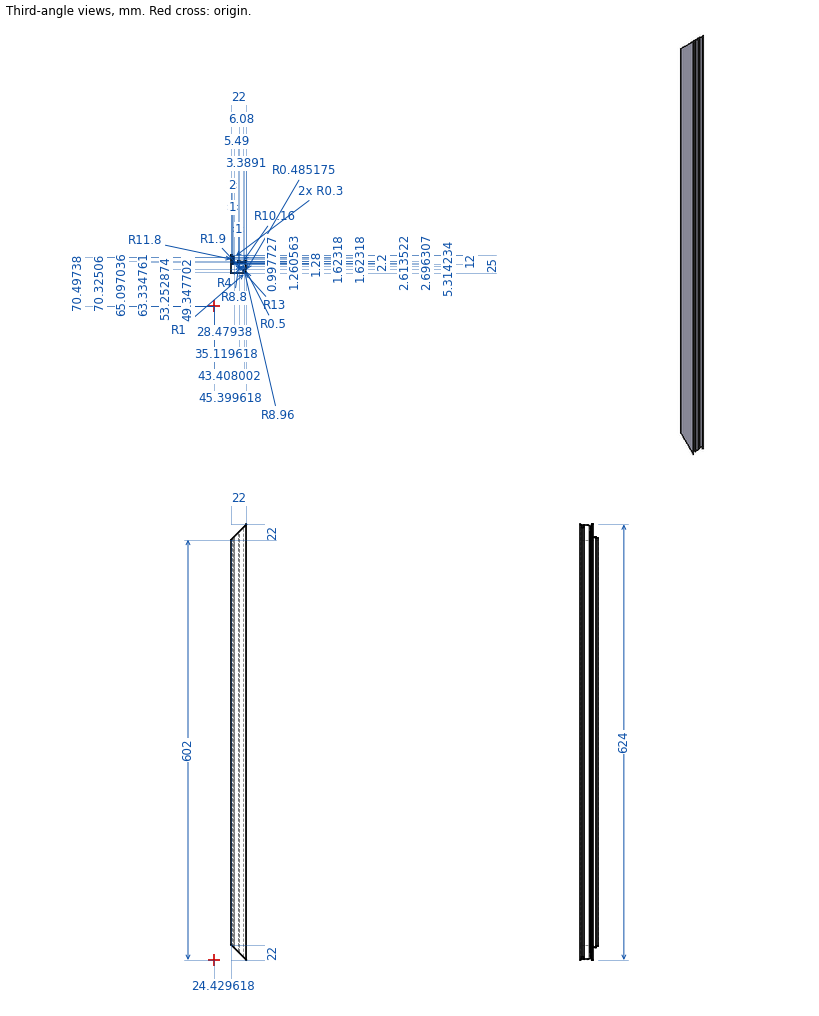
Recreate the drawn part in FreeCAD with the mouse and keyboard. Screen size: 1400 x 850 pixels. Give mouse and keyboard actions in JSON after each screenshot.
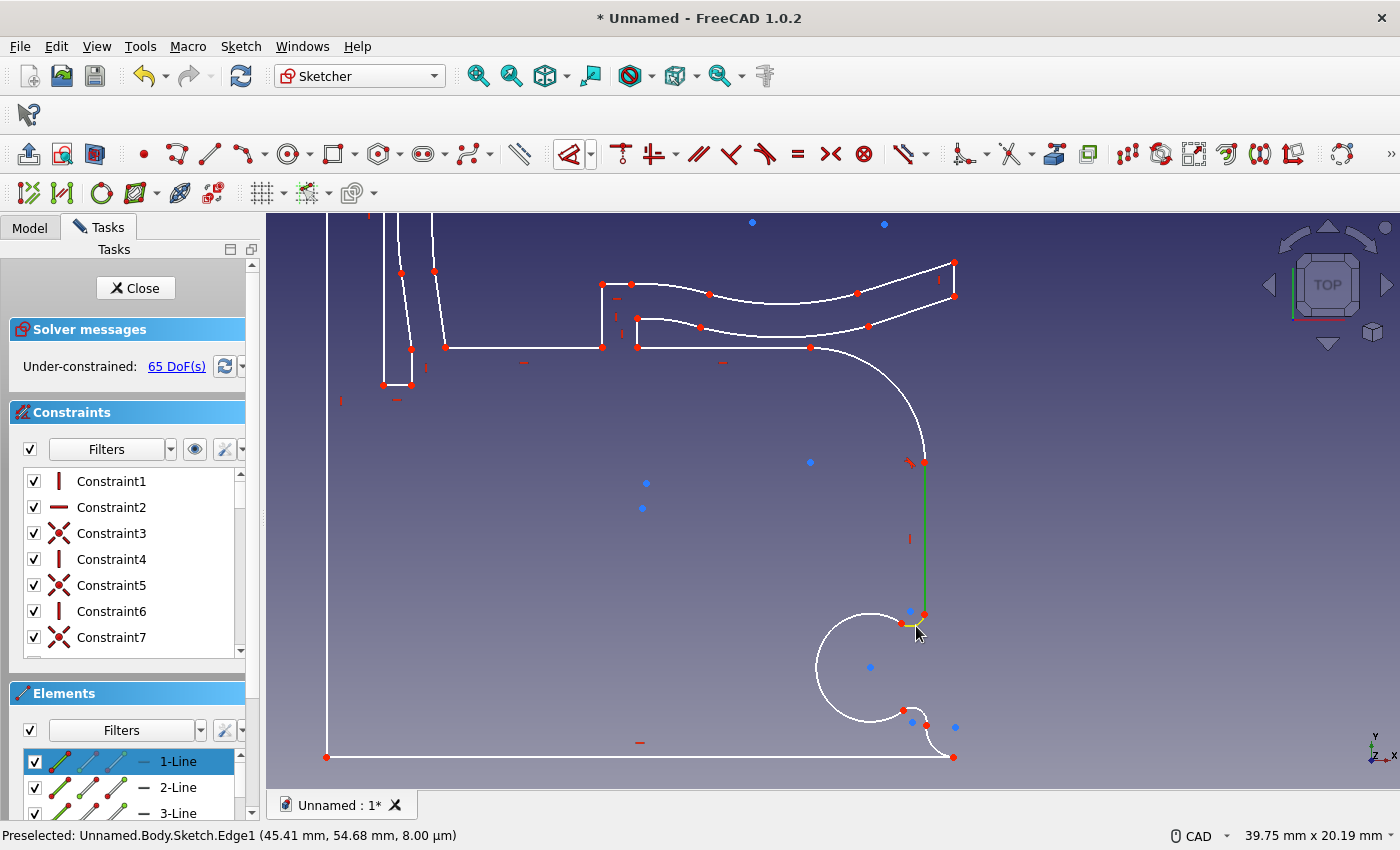
{"action": "left_click", "coordinate": [916, 625]}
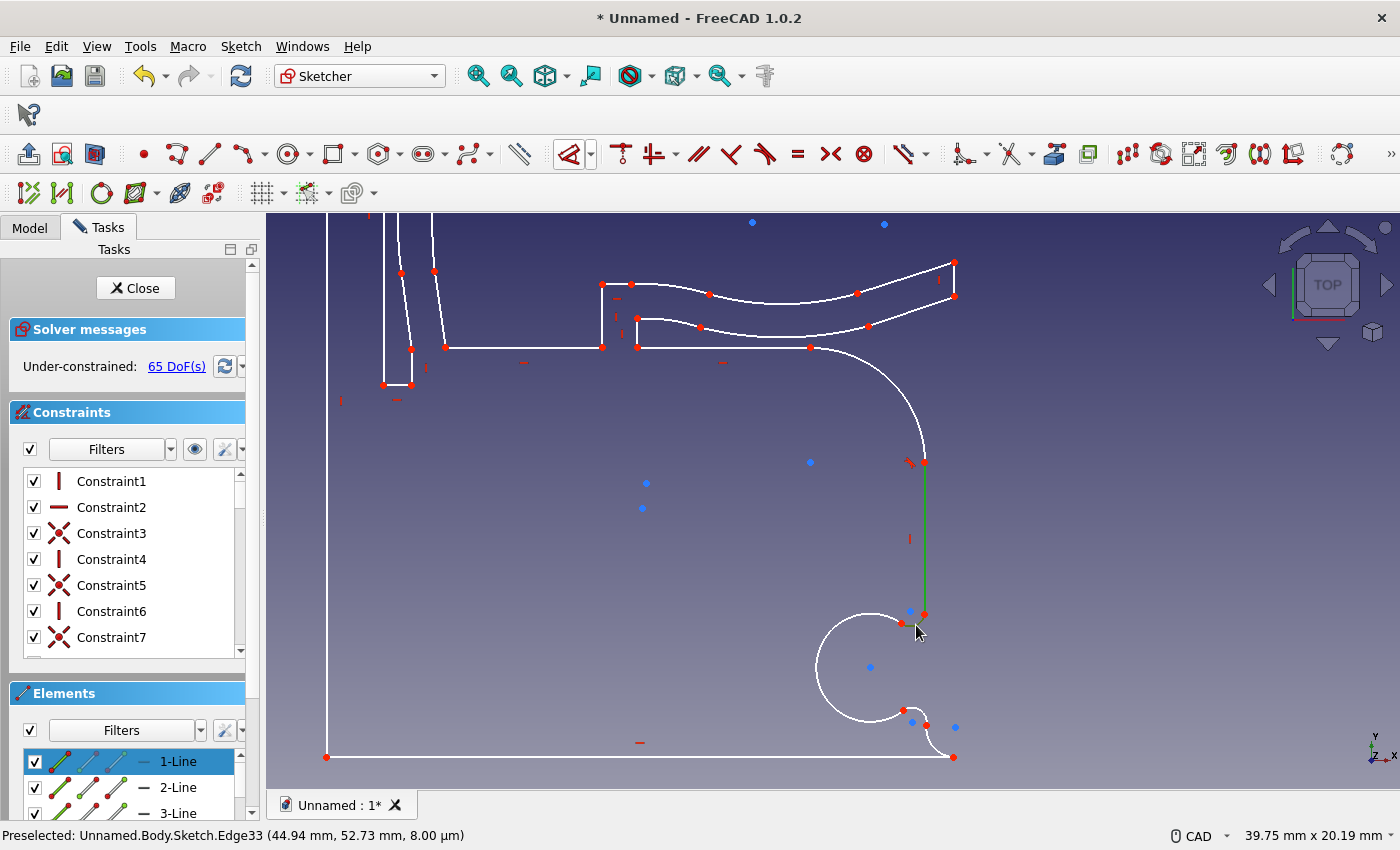
{"action": "key", "text": "t"}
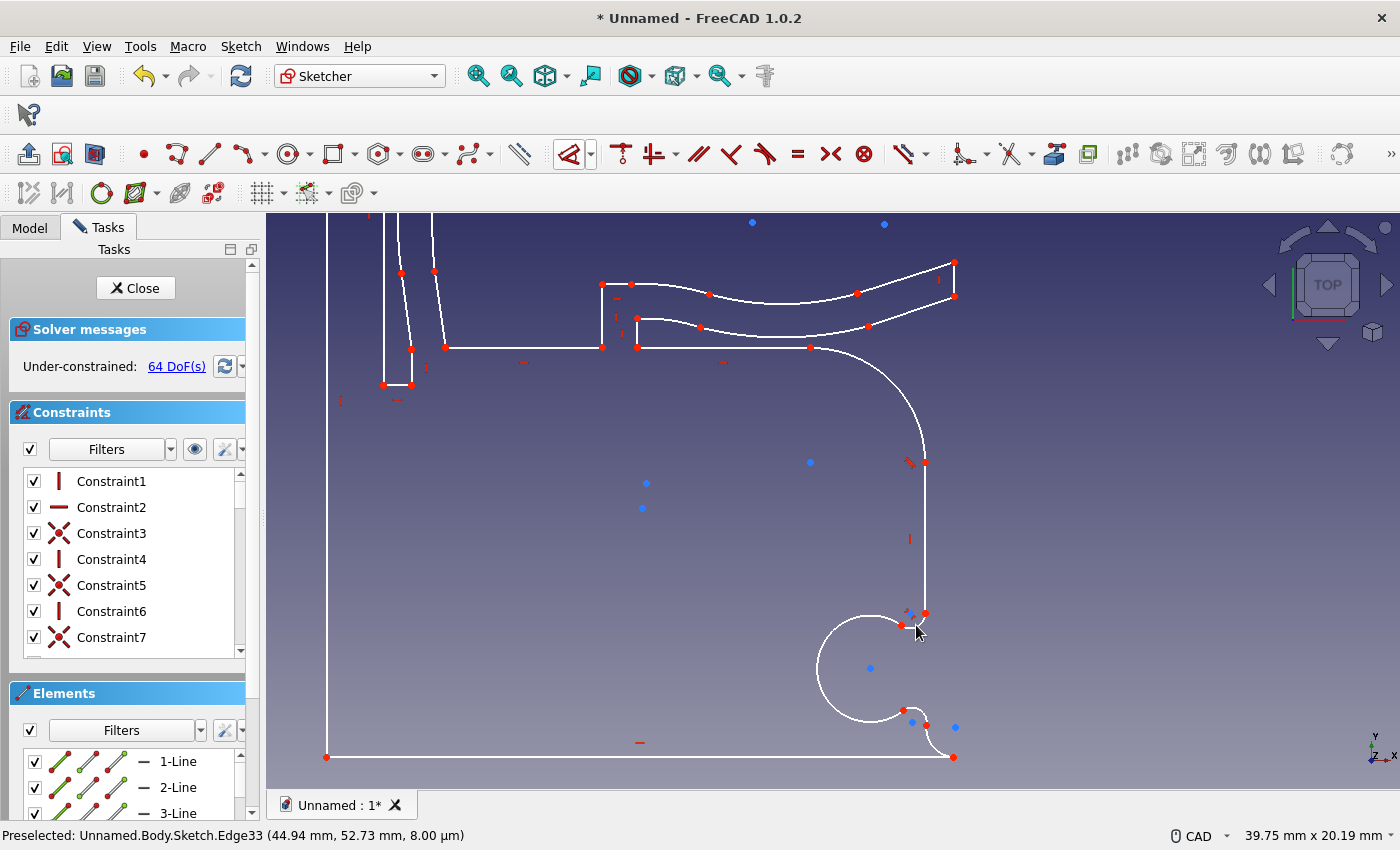
{"action": "left_click", "coordinate": [758, 348]}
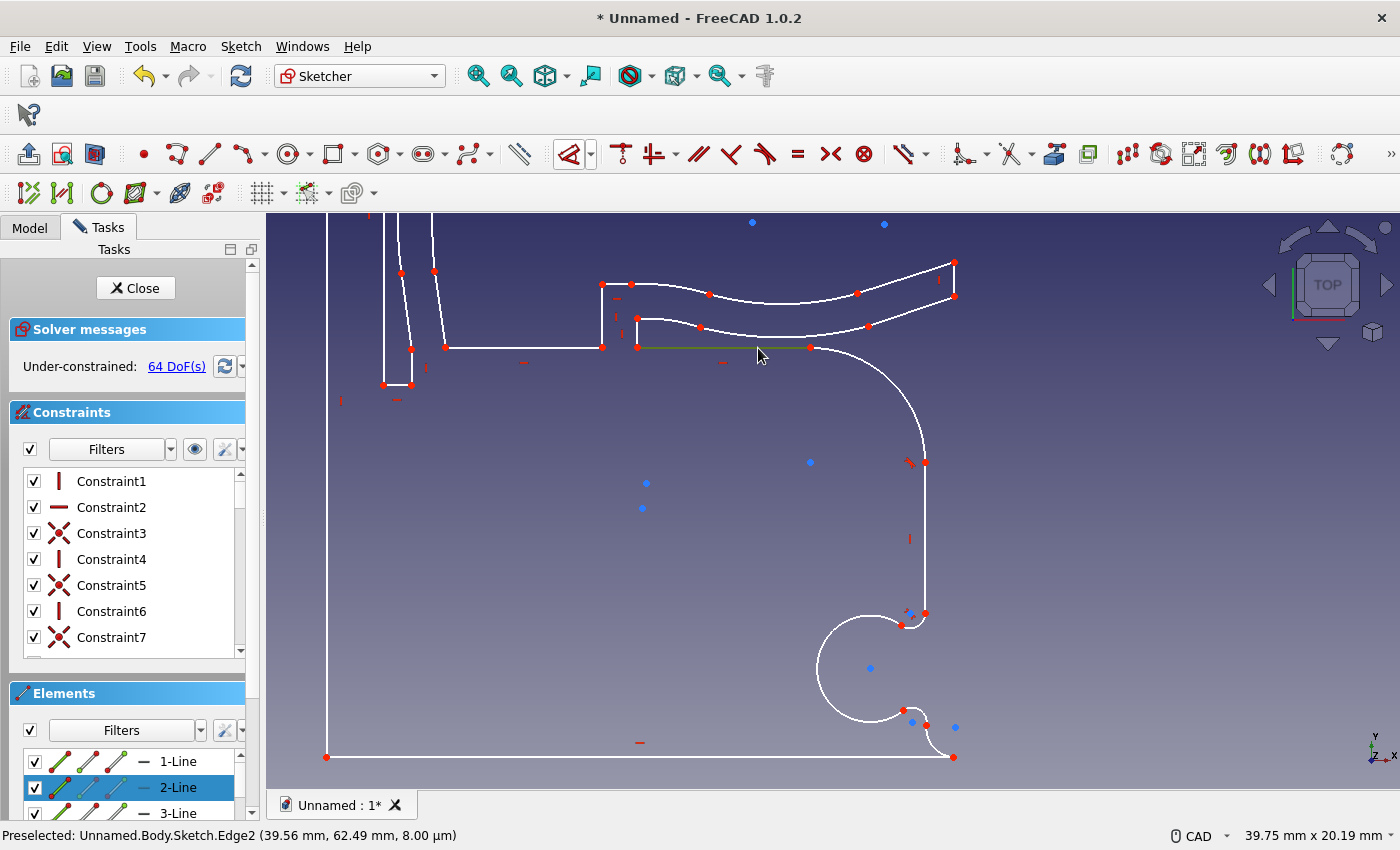
{"action": "left_click", "coordinate": [913, 410]}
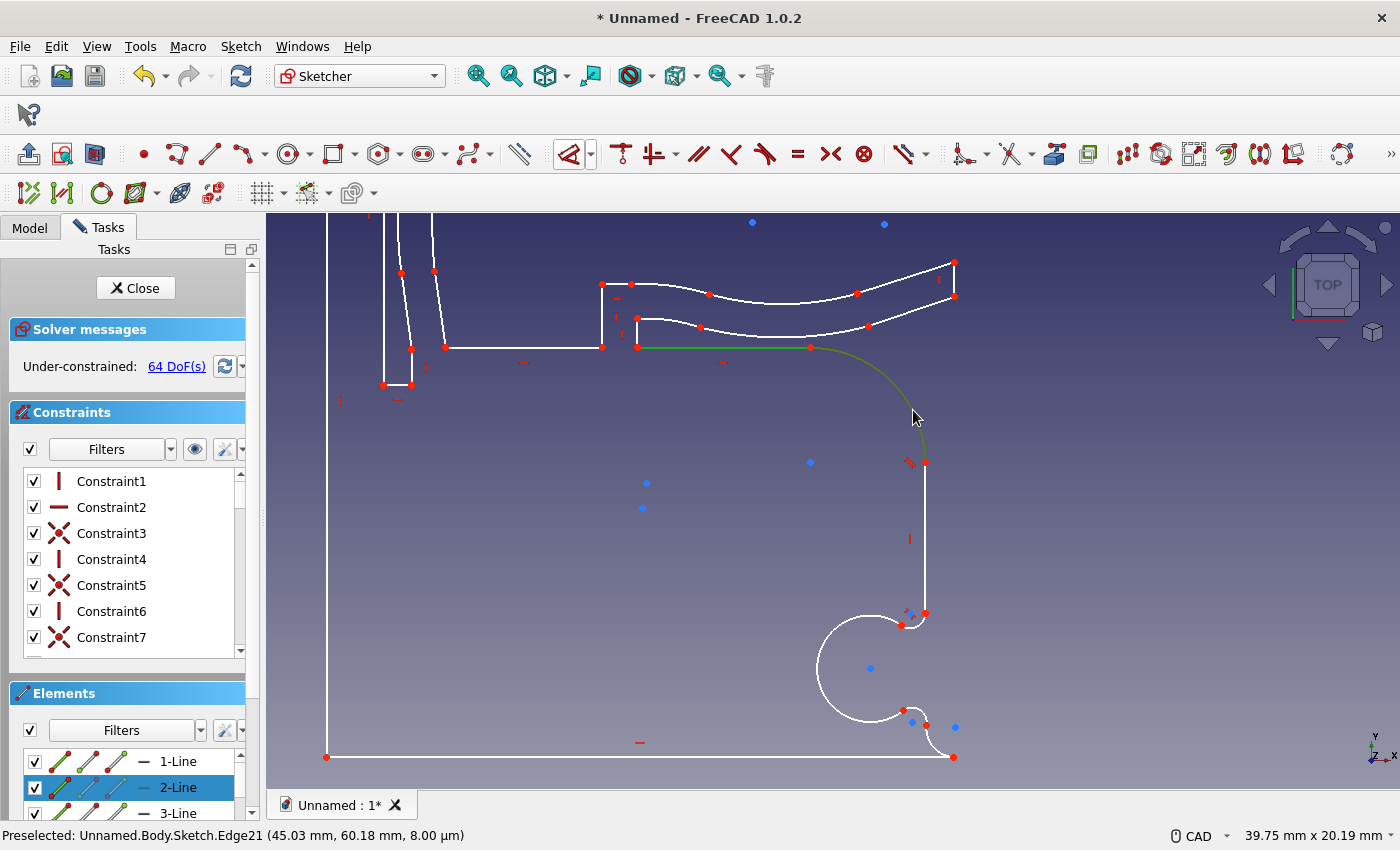
{"action": "key", "text": "t"}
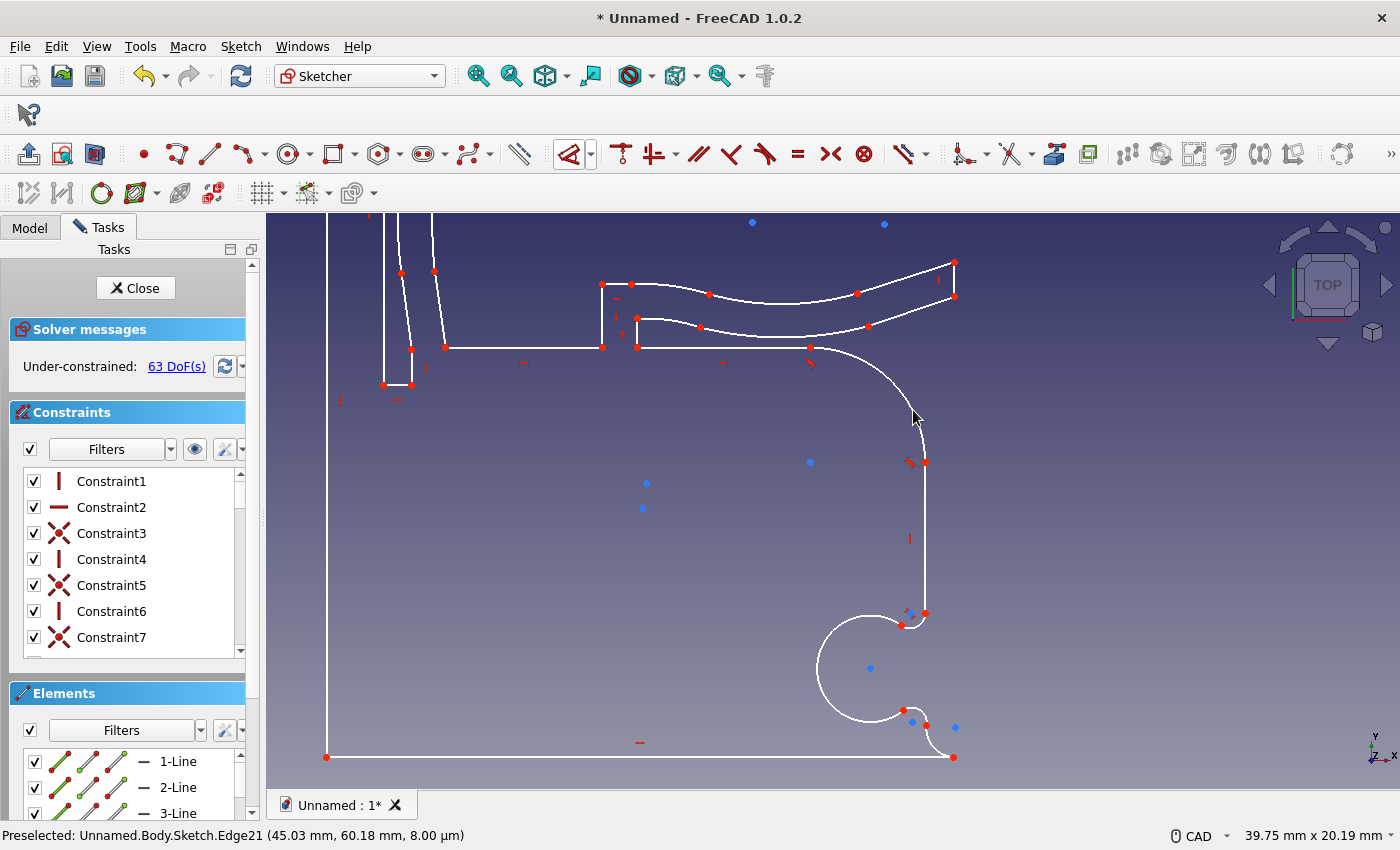
{"action": "left_click", "coordinate": [894, 317]}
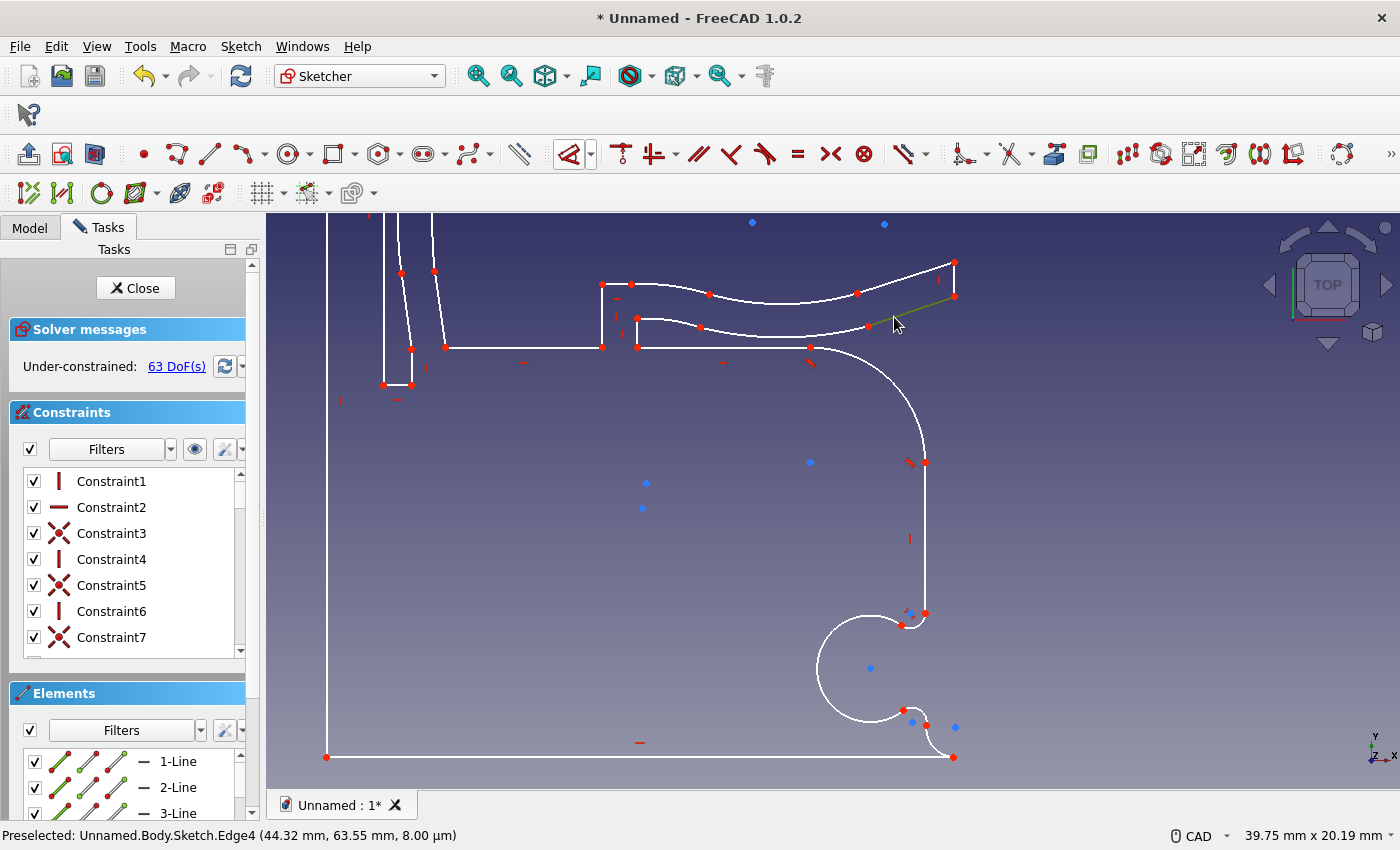
{"action": "left_click", "coordinate": [750, 336]}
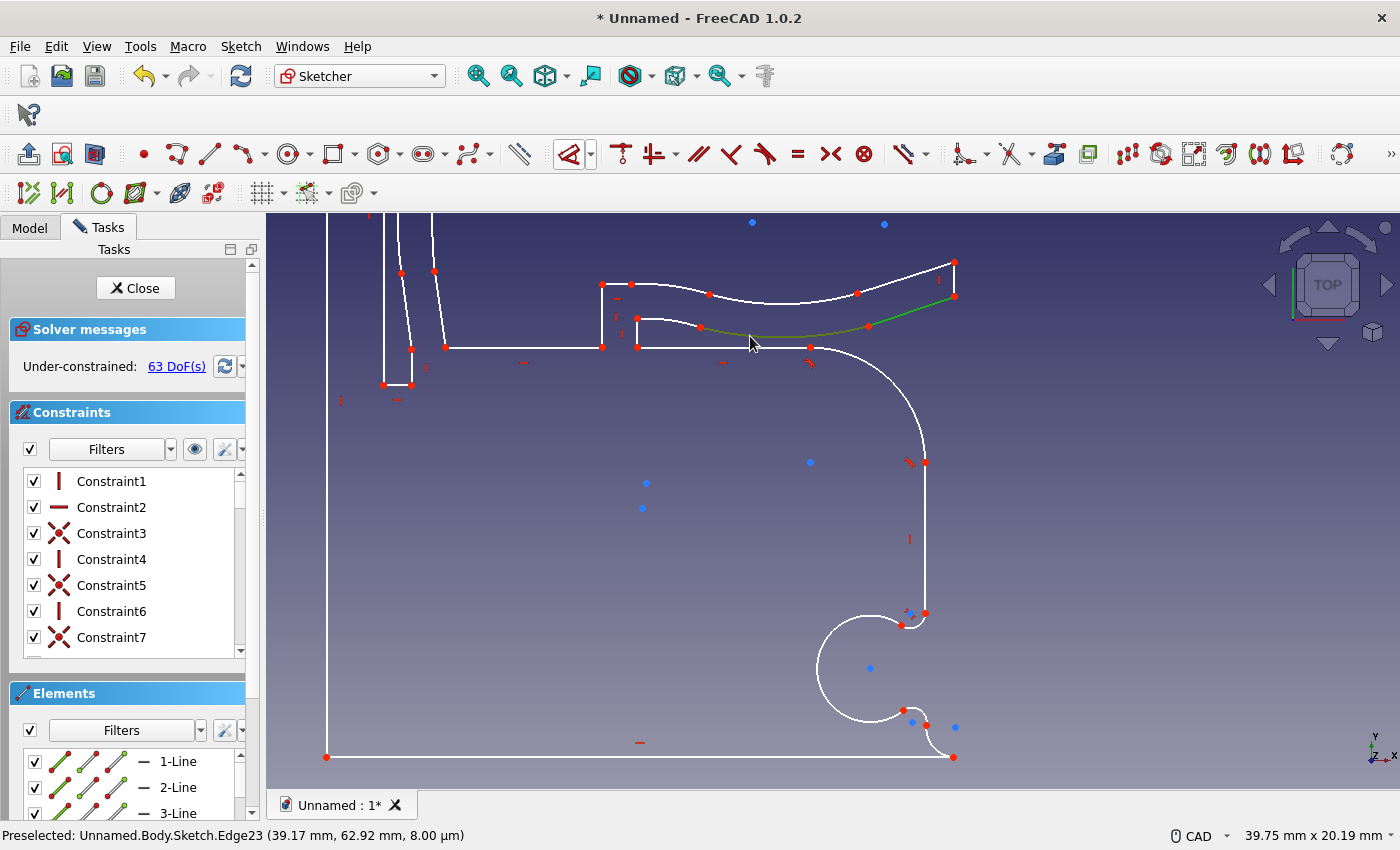
{"action": "key", "text": "t"}